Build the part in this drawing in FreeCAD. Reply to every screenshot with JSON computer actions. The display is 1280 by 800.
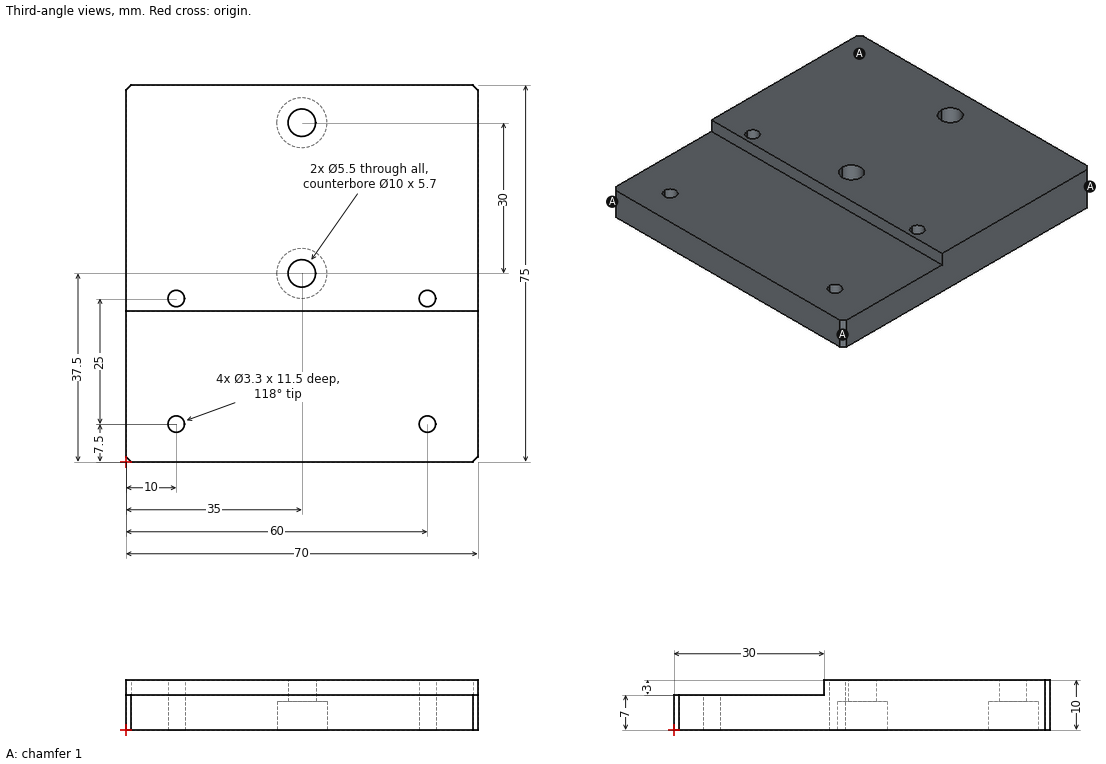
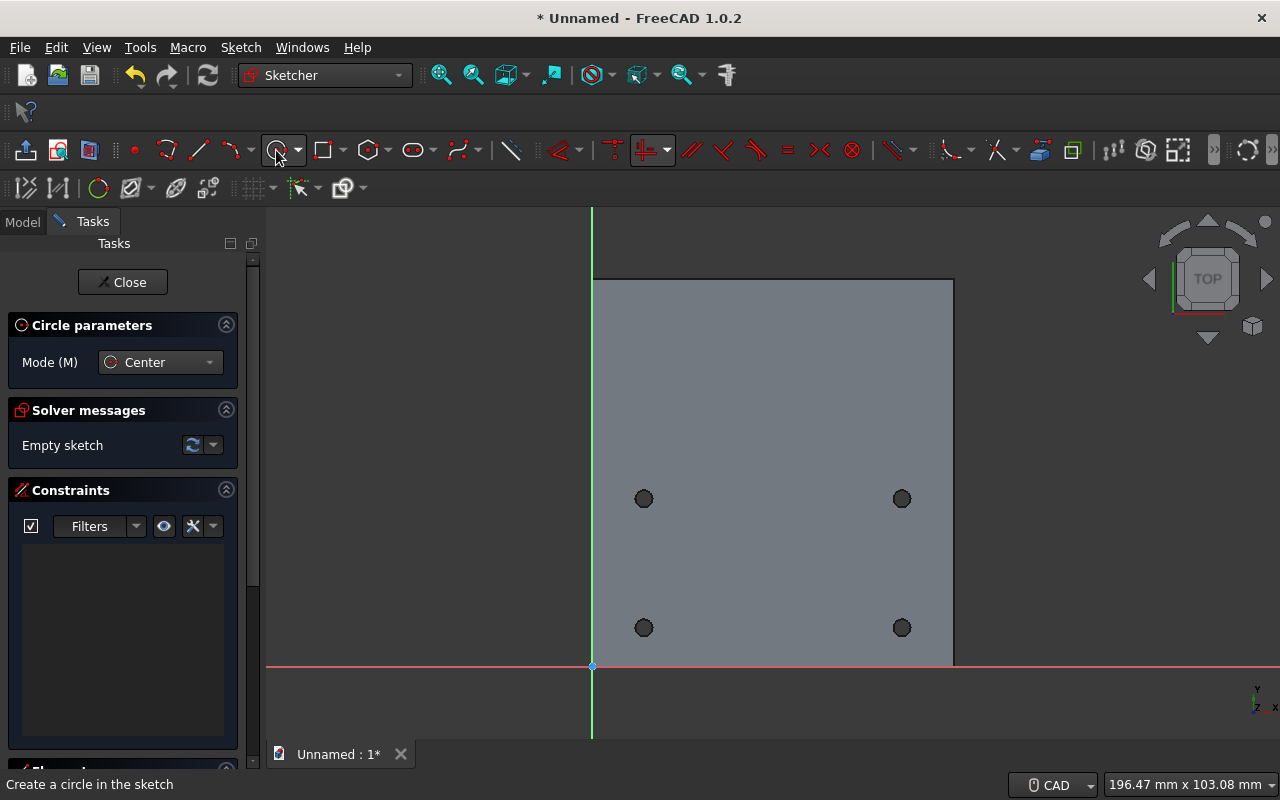
{"action": "scroll", "coordinate": [773, 473], "scroll_direction": "up", "scroll_amount": 3}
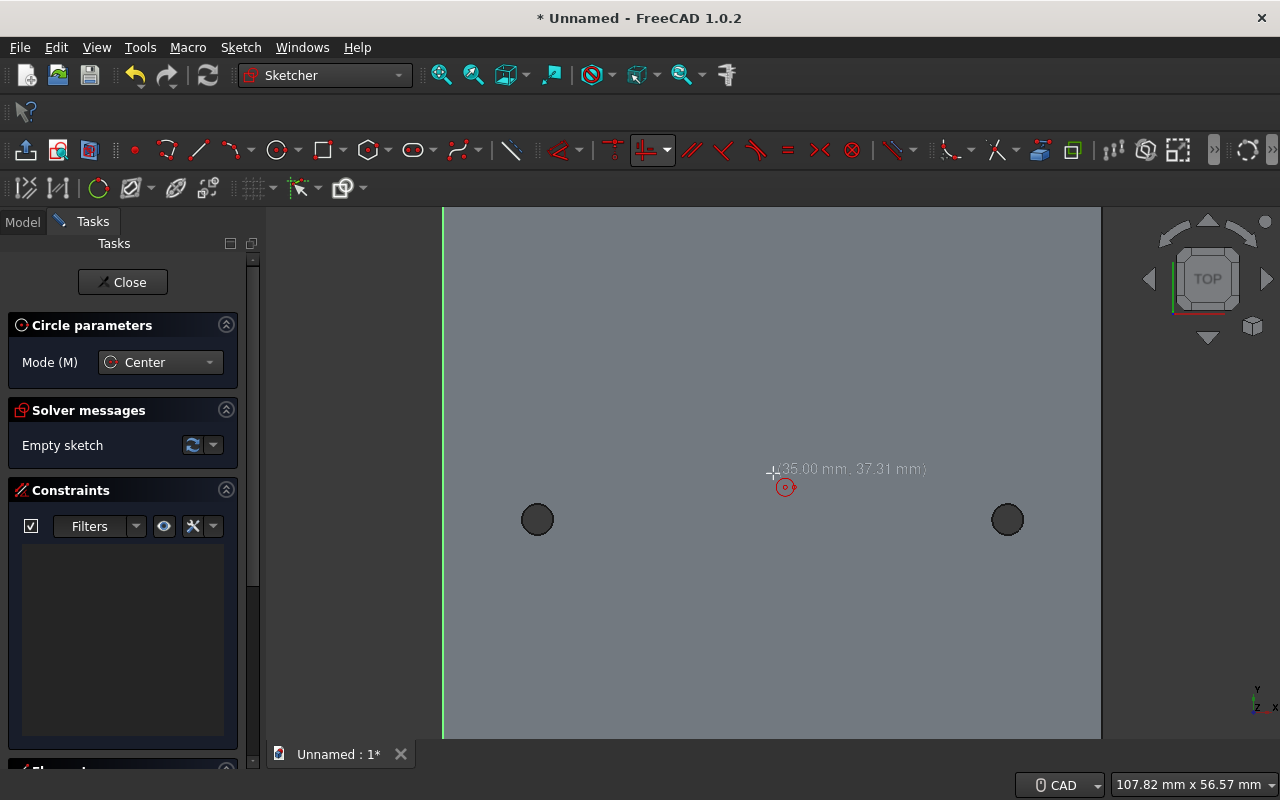
{"action": "left_click", "coordinate": [773, 473]}
{"action": "mouse_move", "coordinate": [791, 454]}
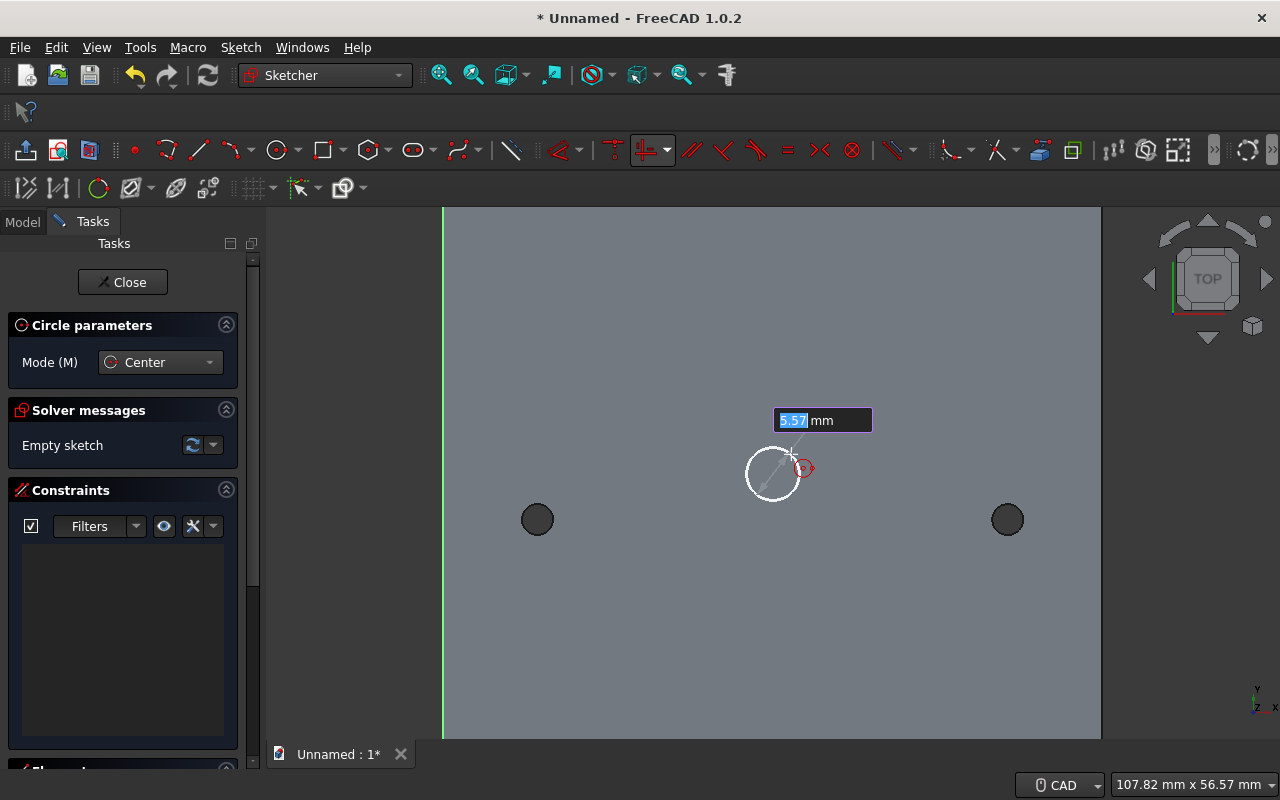
{"action": "type", "text": "5.5"}
{"action": "key", "text": "Return"}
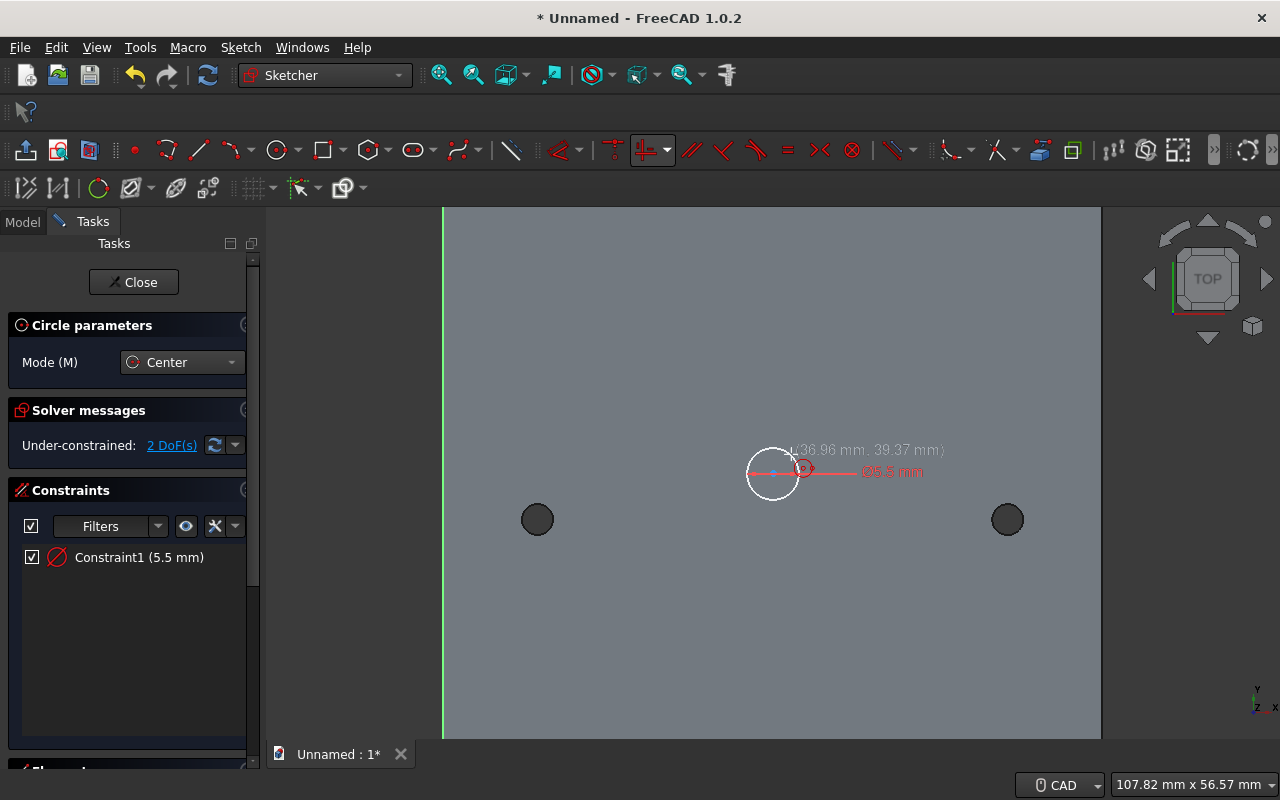
{"action": "scroll", "coordinate": [806, 446], "scroll_direction": "down", "scroll_amount": 3}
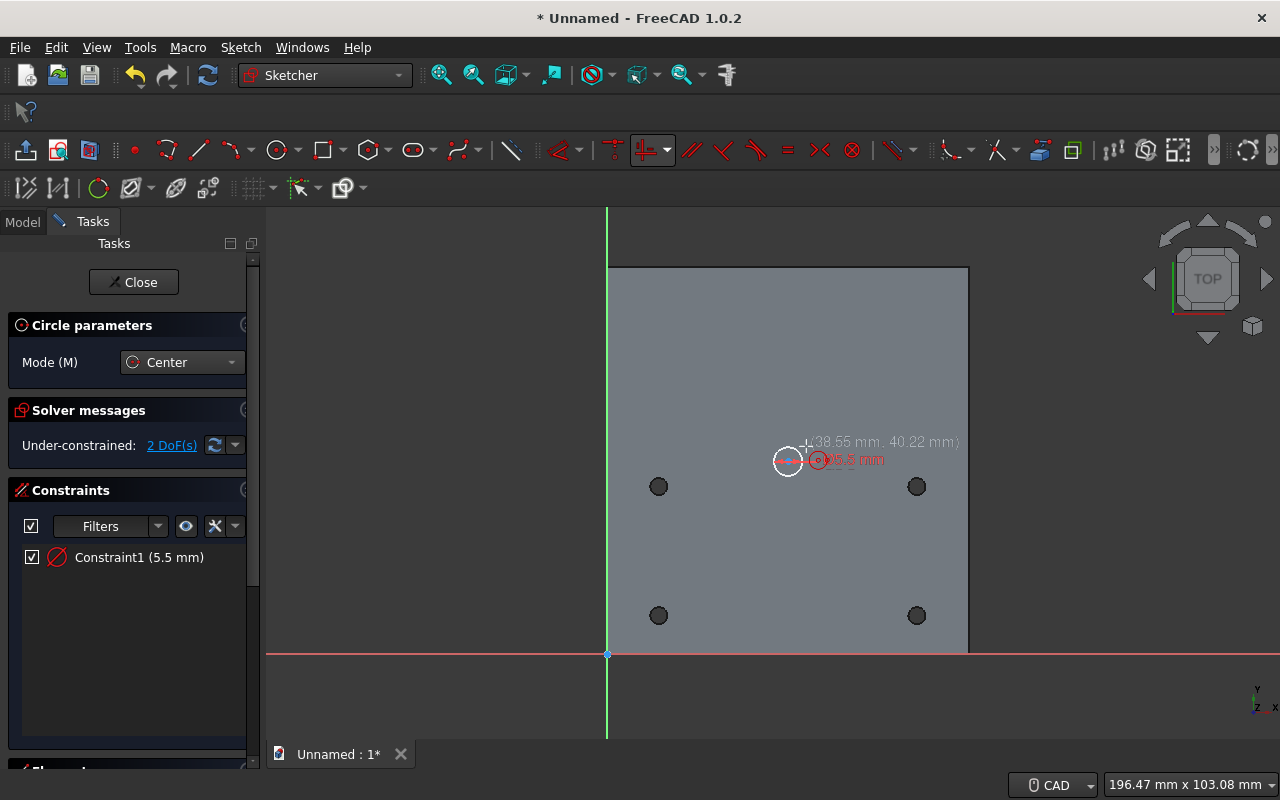
{"action": "scroll", "coordinate": [788, 306], "scroll_direction": "up", "scroll_amount": 3}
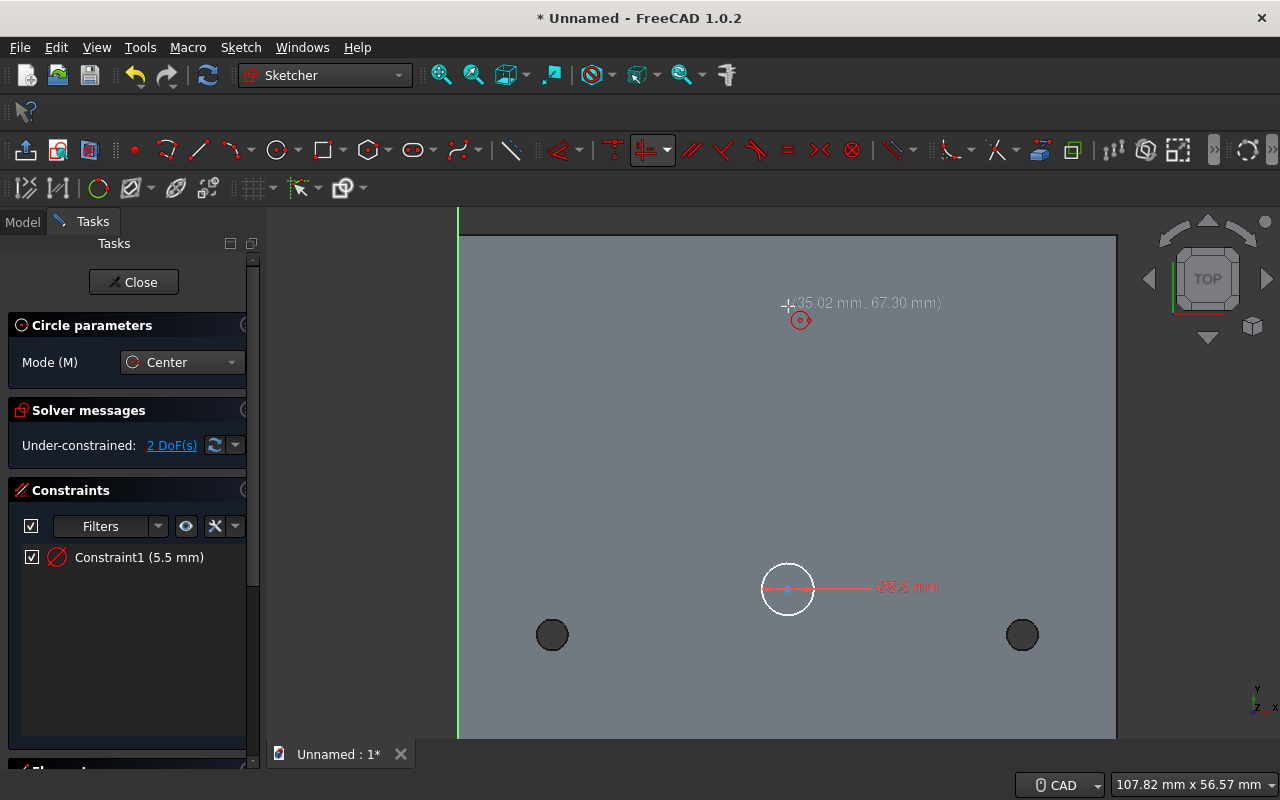
{"action": "left_click", "coordinate": [787, 306]}
{"action": "mouse_move", "coordinate": [806, 287]}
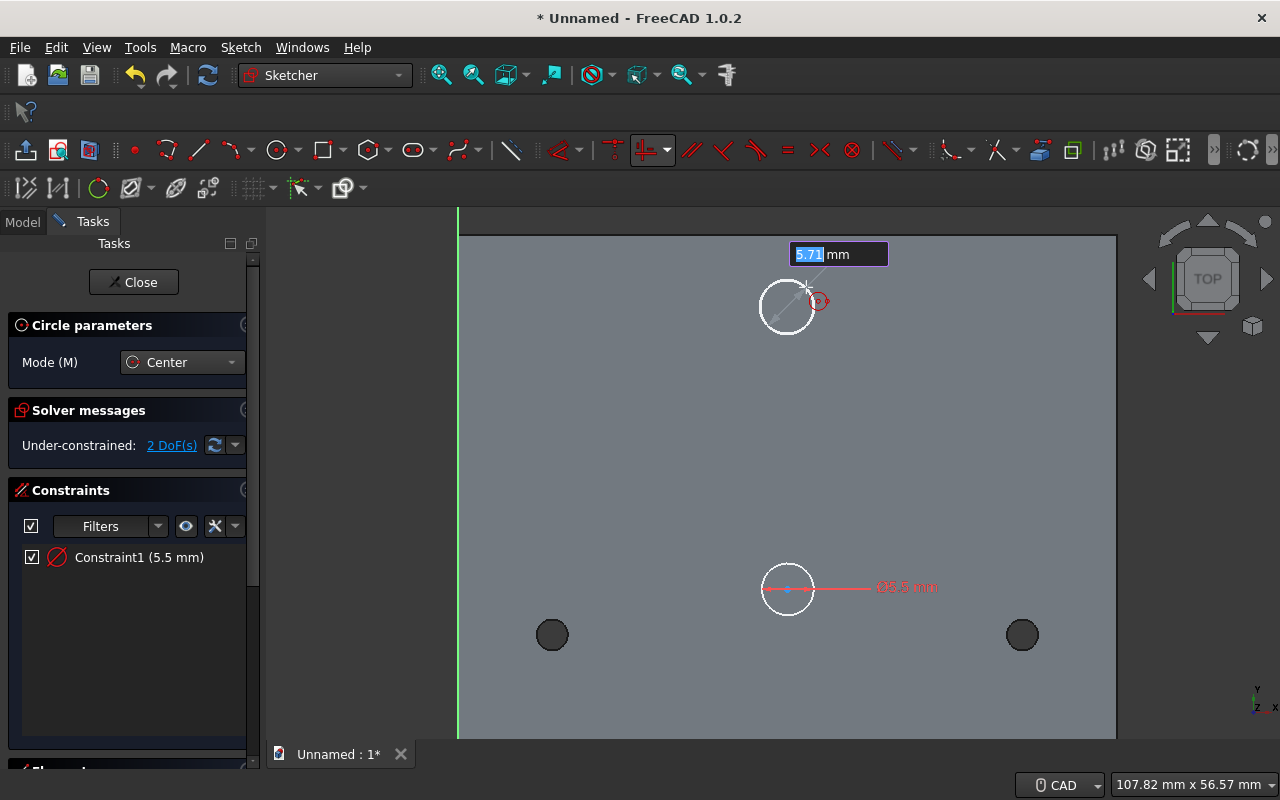
{"action": "type", "text": "5.5"}
{"action": "key", "text": "Return"}
{"action": "key", "text": "Escape"}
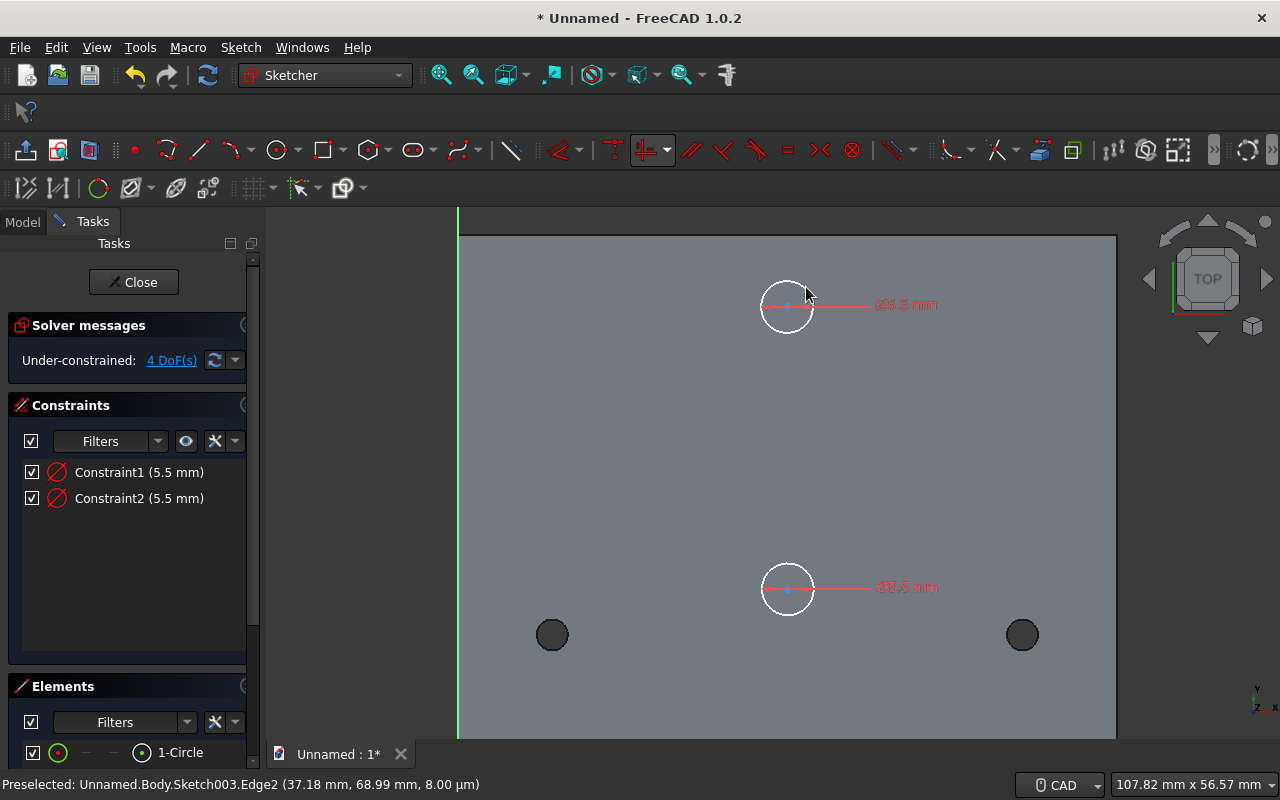
{"action": "left_click", "coordinate": [788, 589]}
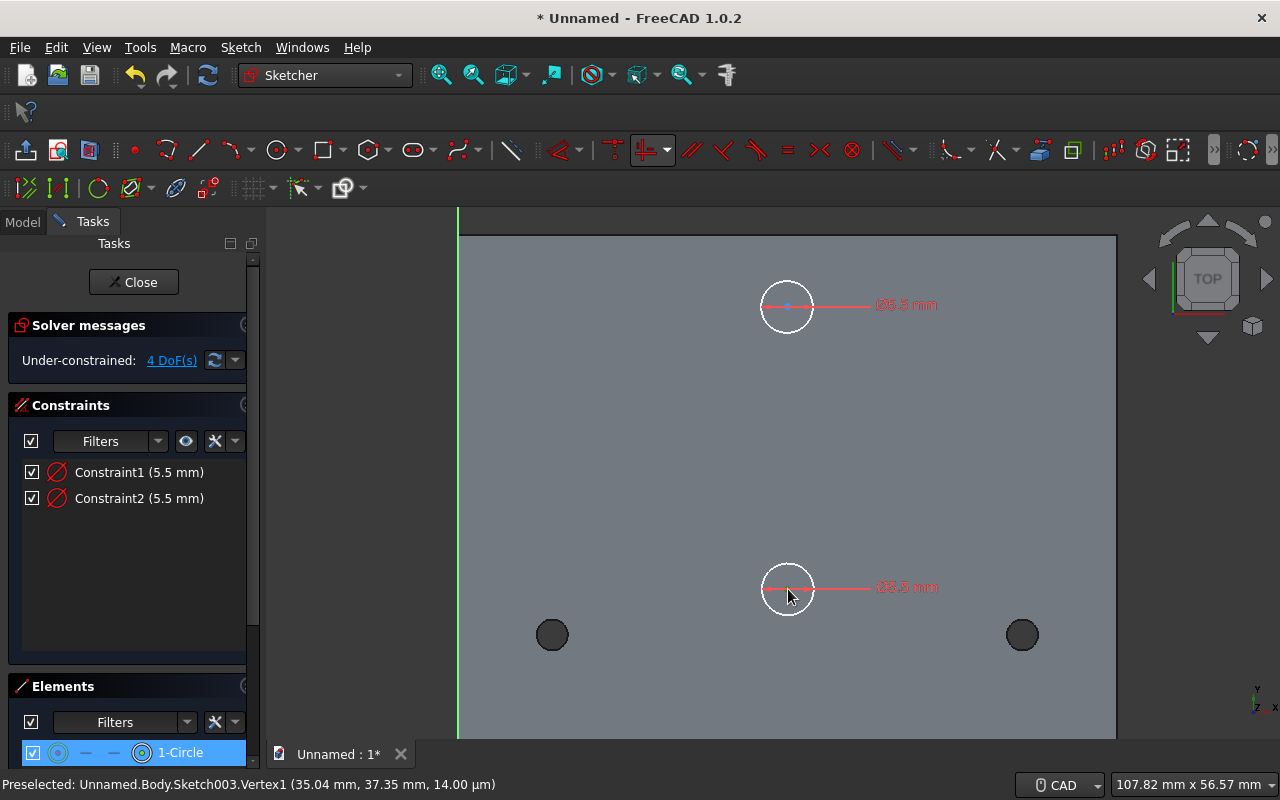
{"action": "left_click", "coordinate": [787, 307]}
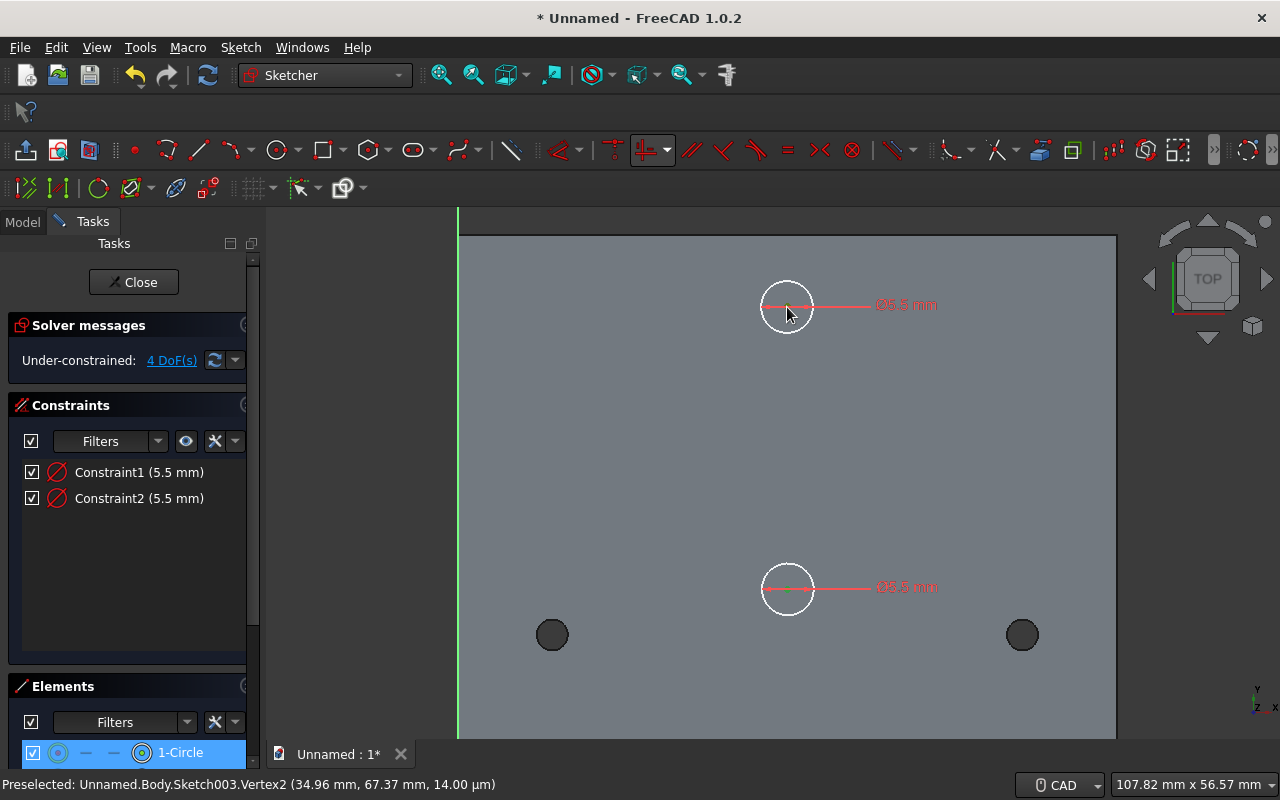
{"action": "key", "text": "v"}